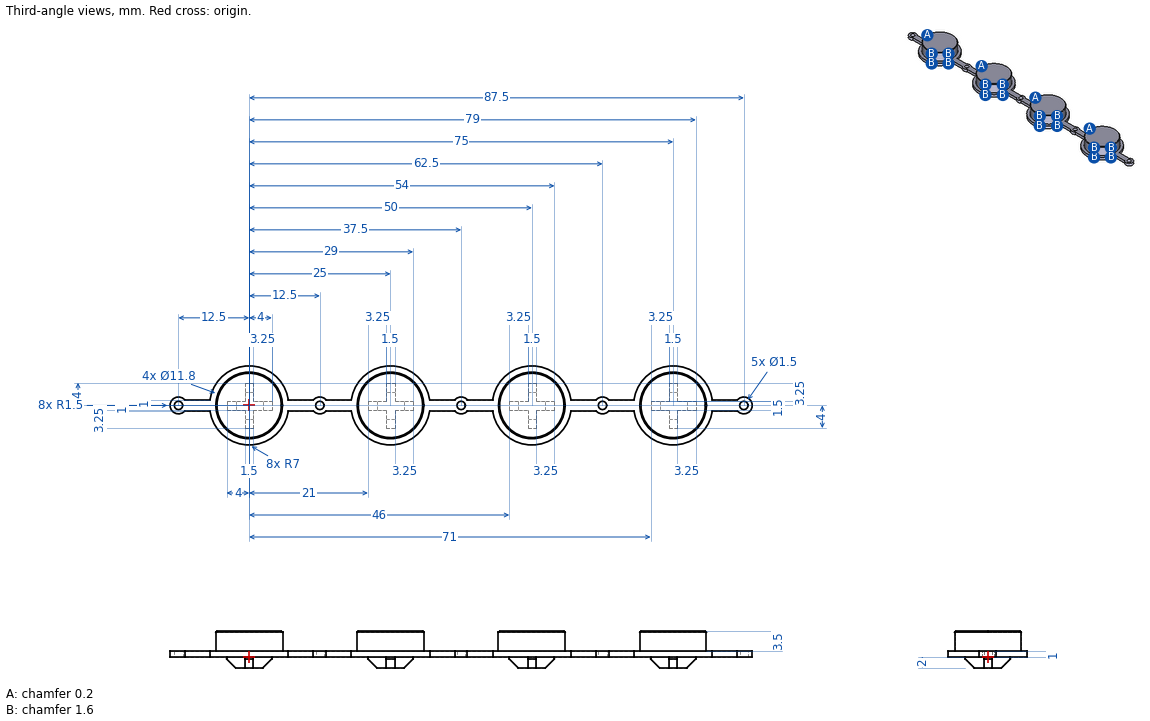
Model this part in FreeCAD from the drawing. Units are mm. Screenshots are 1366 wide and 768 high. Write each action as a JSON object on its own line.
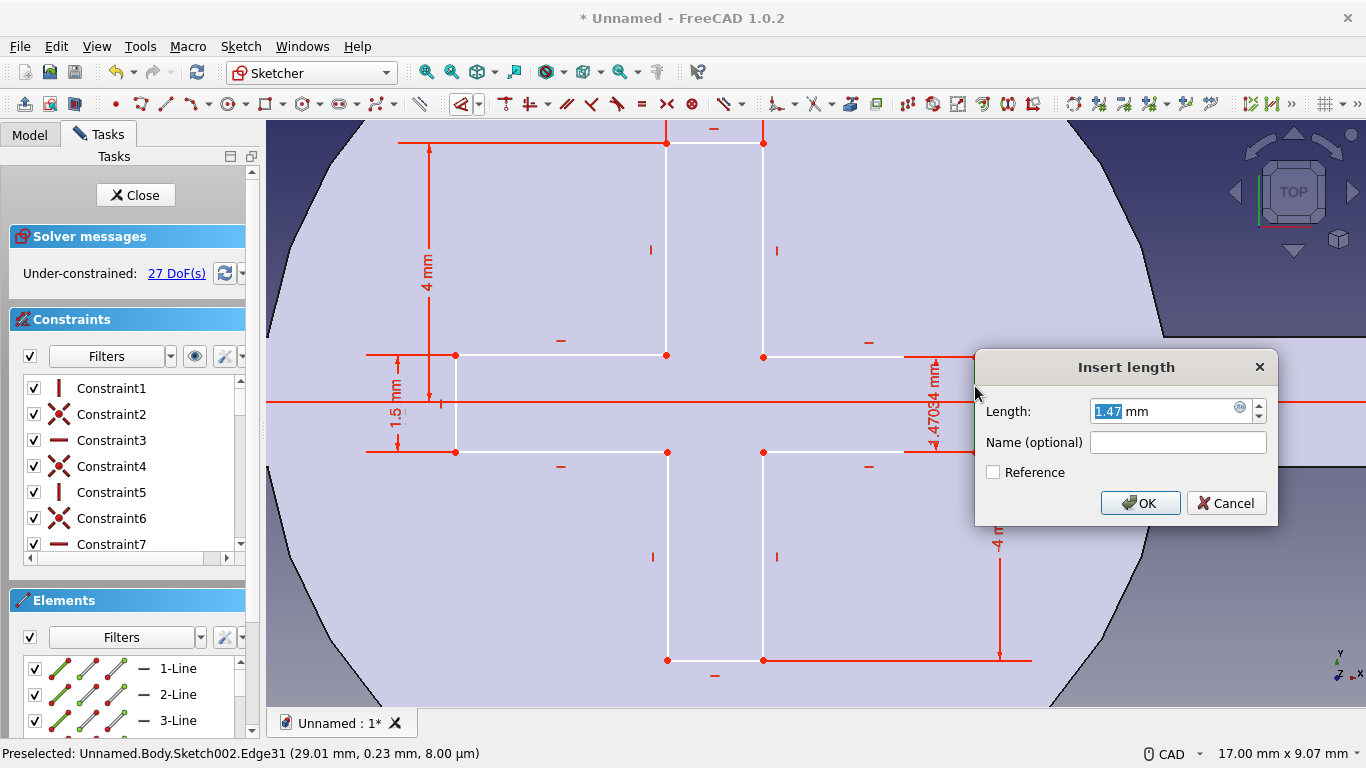
{"action": "type", "text": "1.5"}
{"action": "key", "text": "Return"}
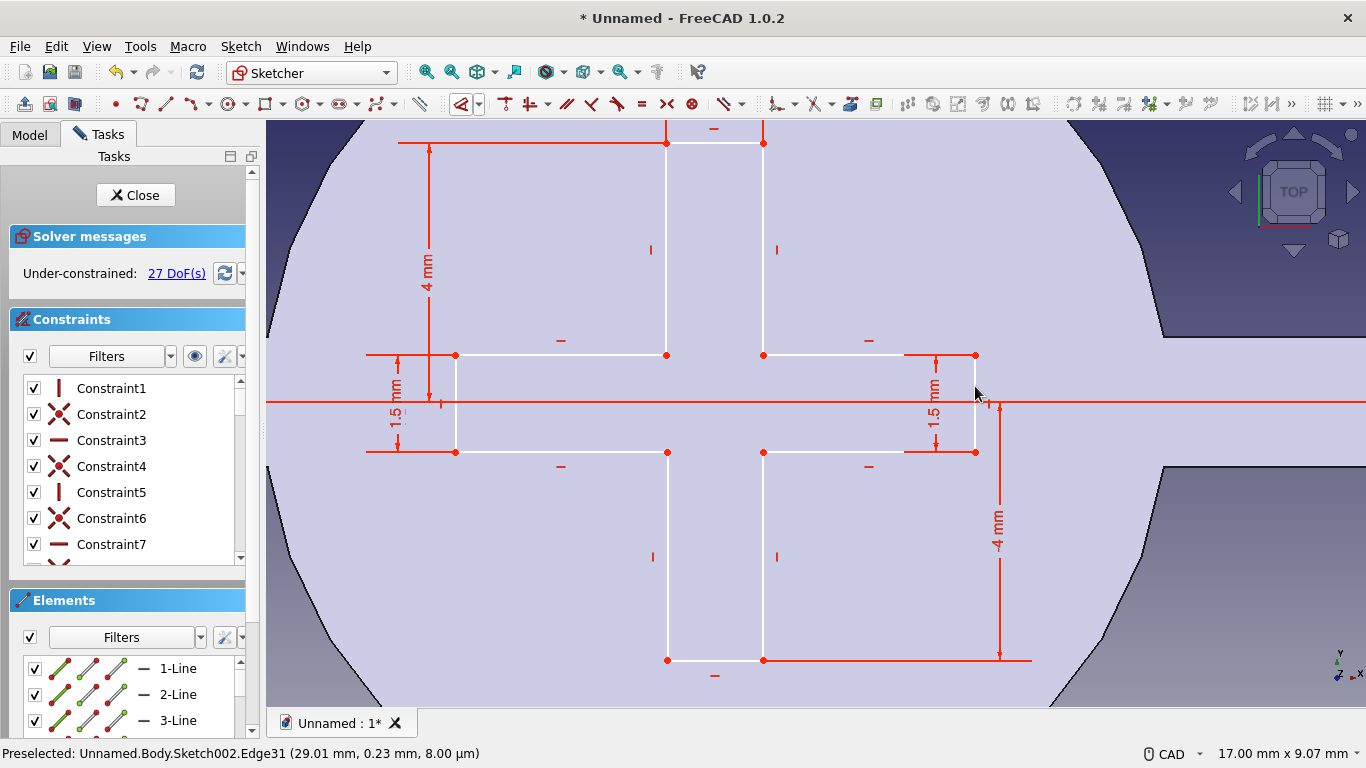
{"action": "left_click", "coordinate": [735, 661]}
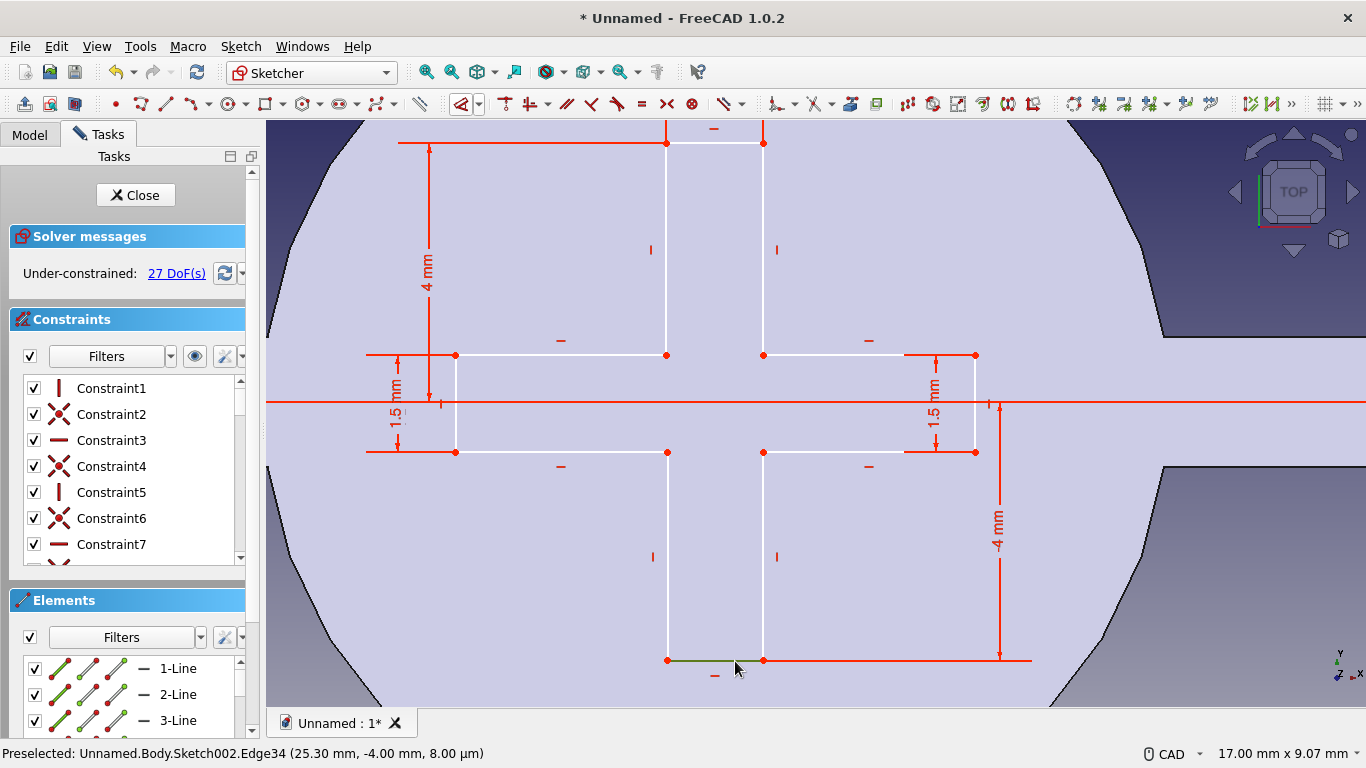
{"action": "key", "text": "l"}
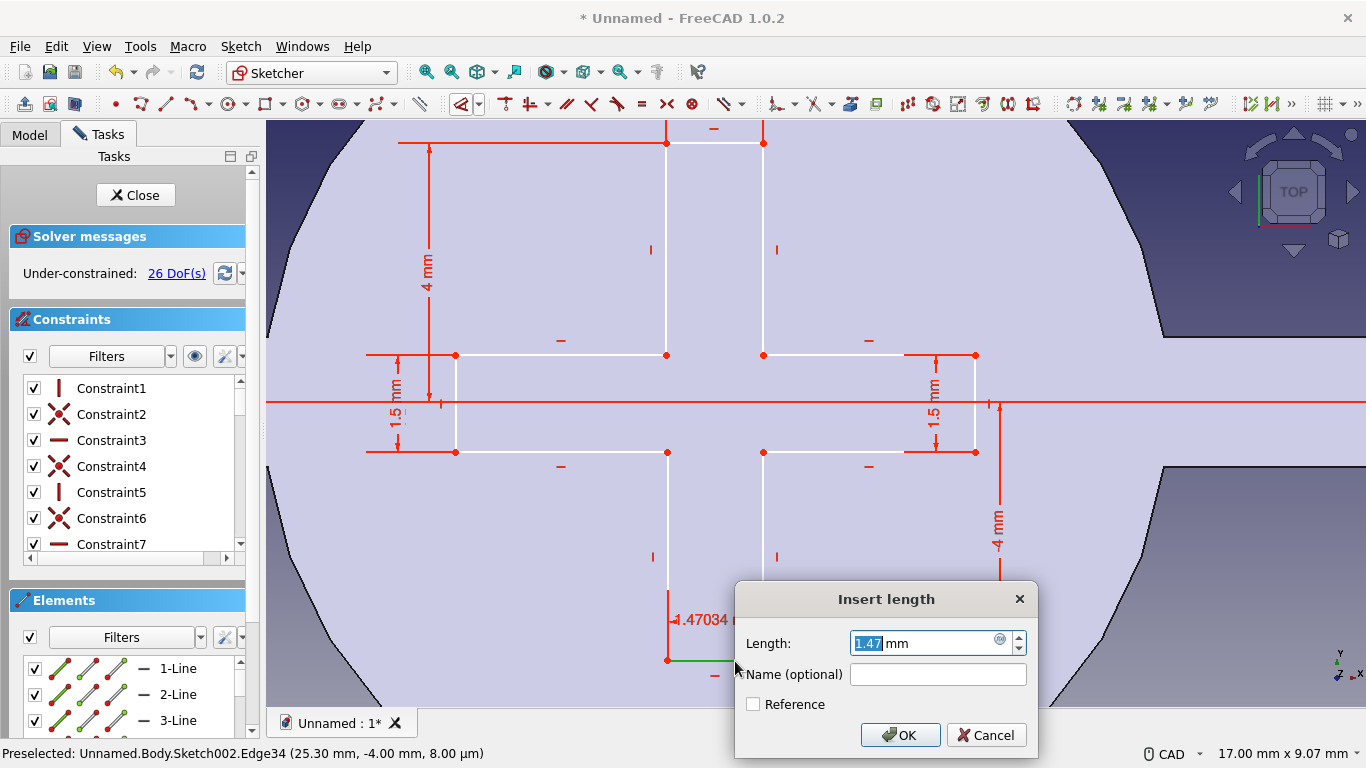
{"action": "type", "text": "1.5"}
{"action": "key", "text": "Return"}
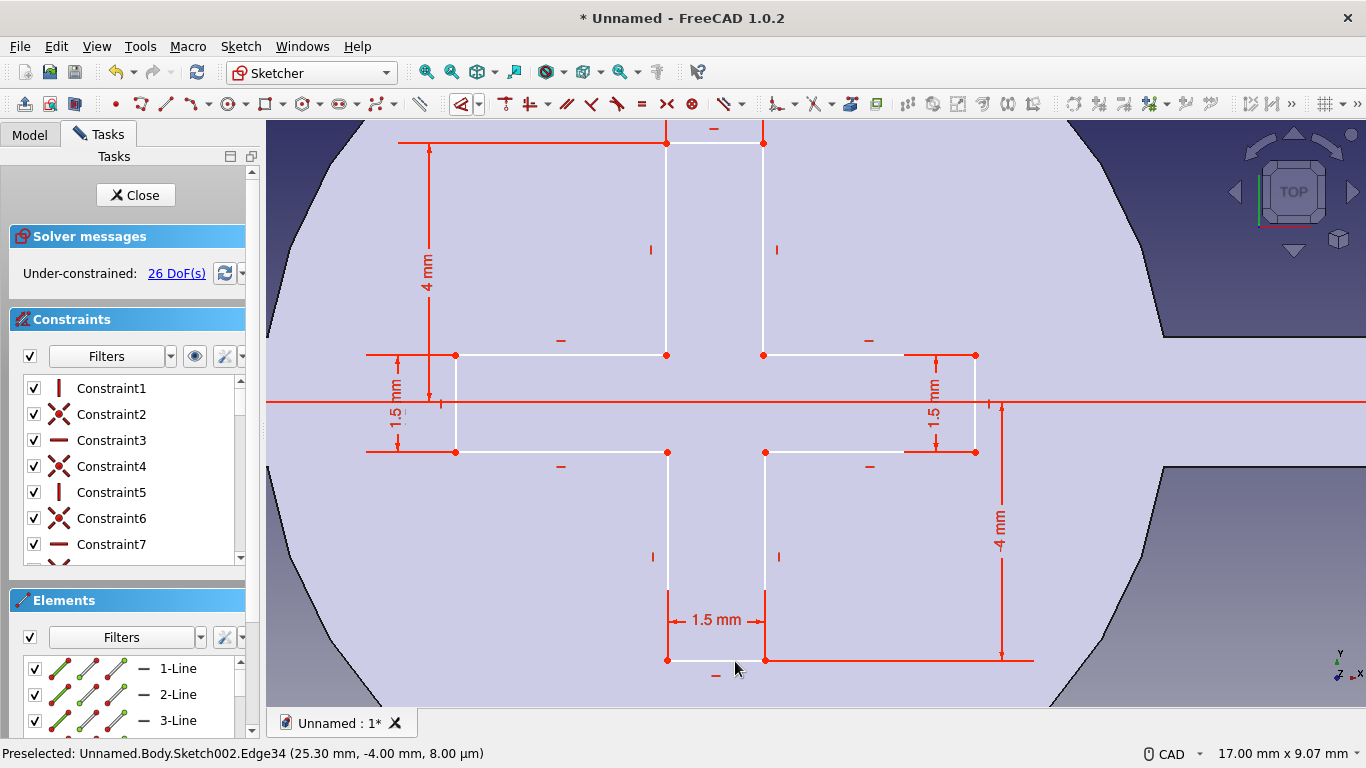
{"action": "scroll", "coordinate": [651, 415], "scroll_direction": "down", "scroll_amount": 11}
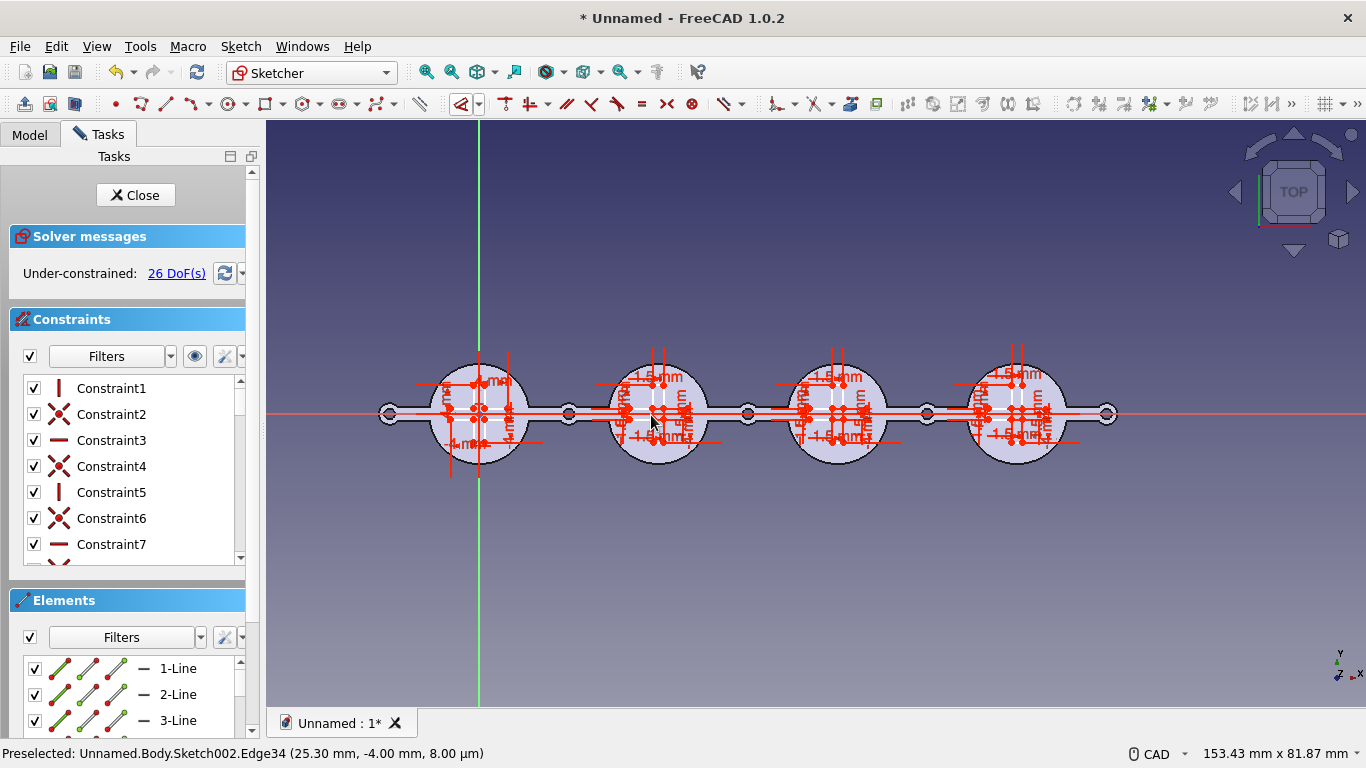
{"action": "scroll", "coordinate": [508, 412], "scroll_direction": "up", "scroll_amount": 10}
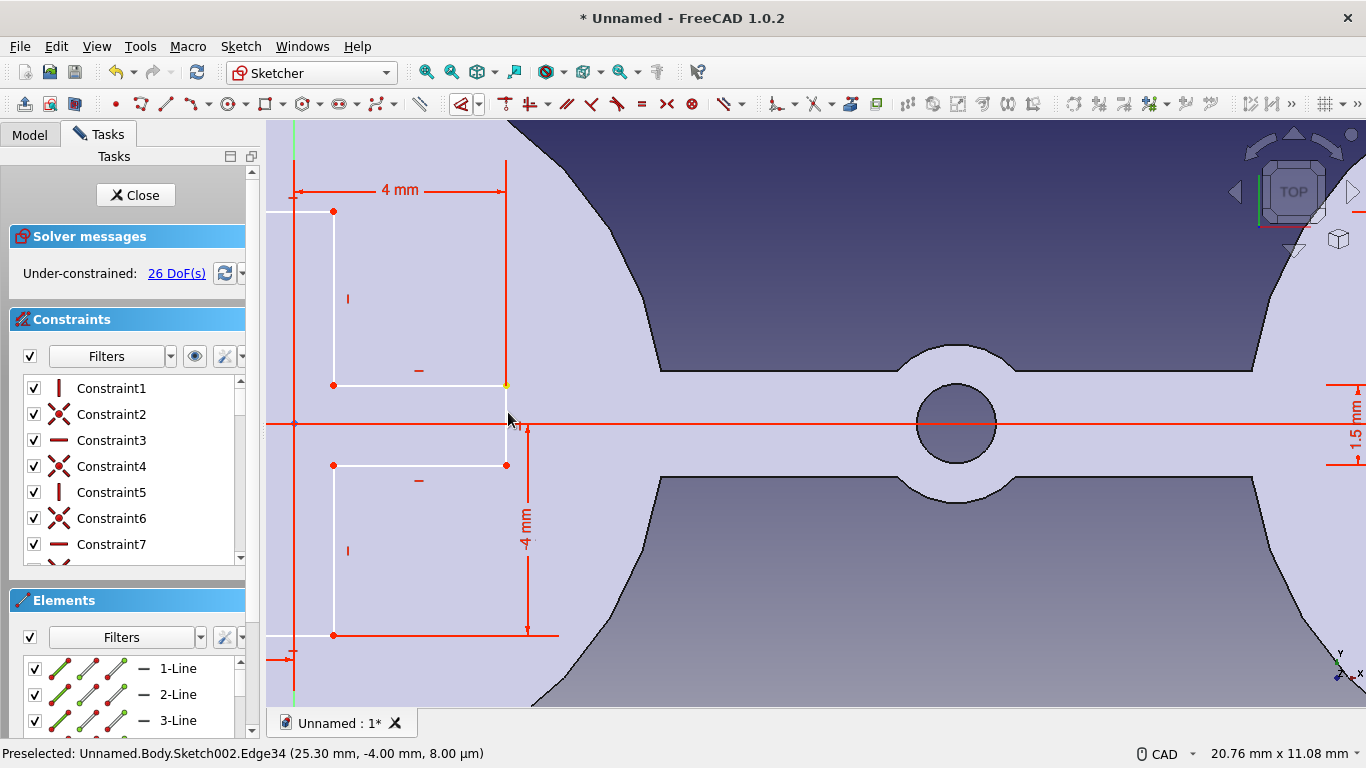
{"action": "left_click", "coordinate": [506, 410]}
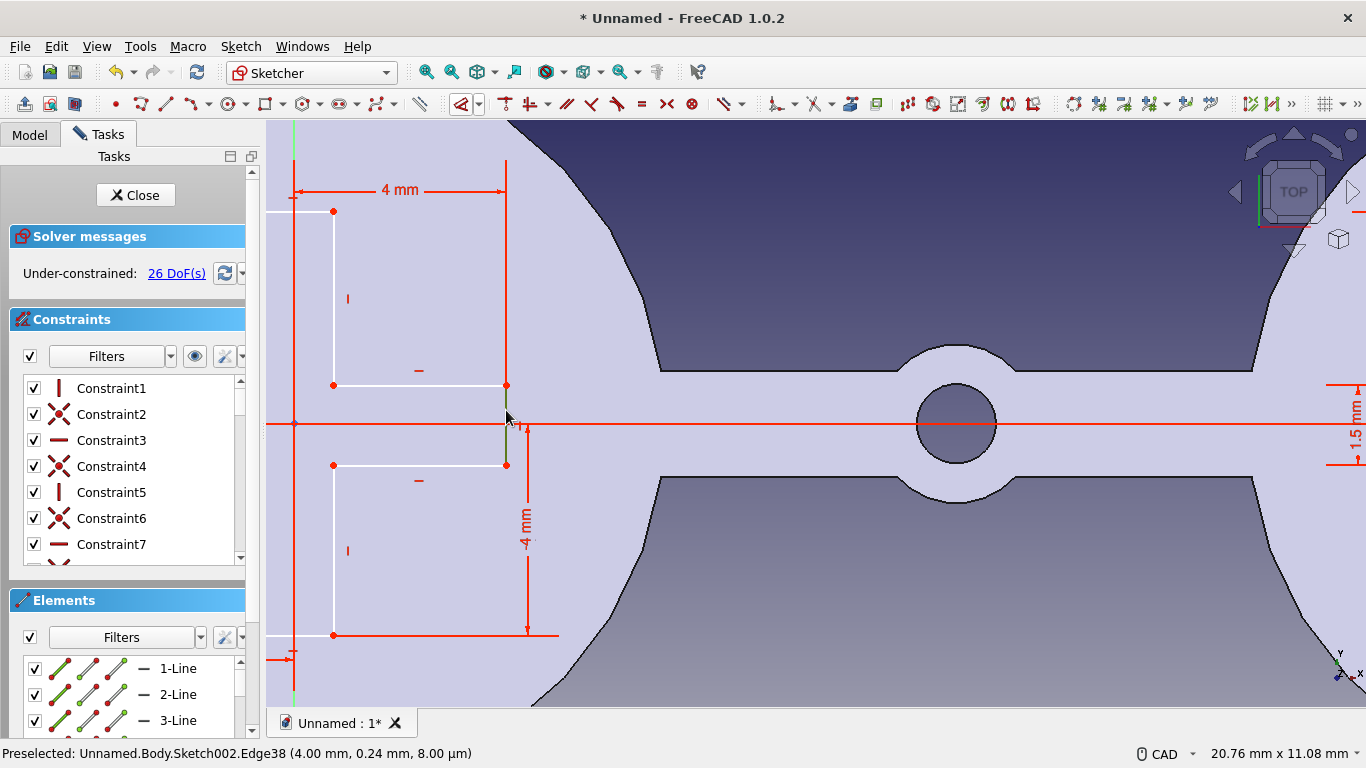
{"action": "left_click", "coordinate": [478, 104]}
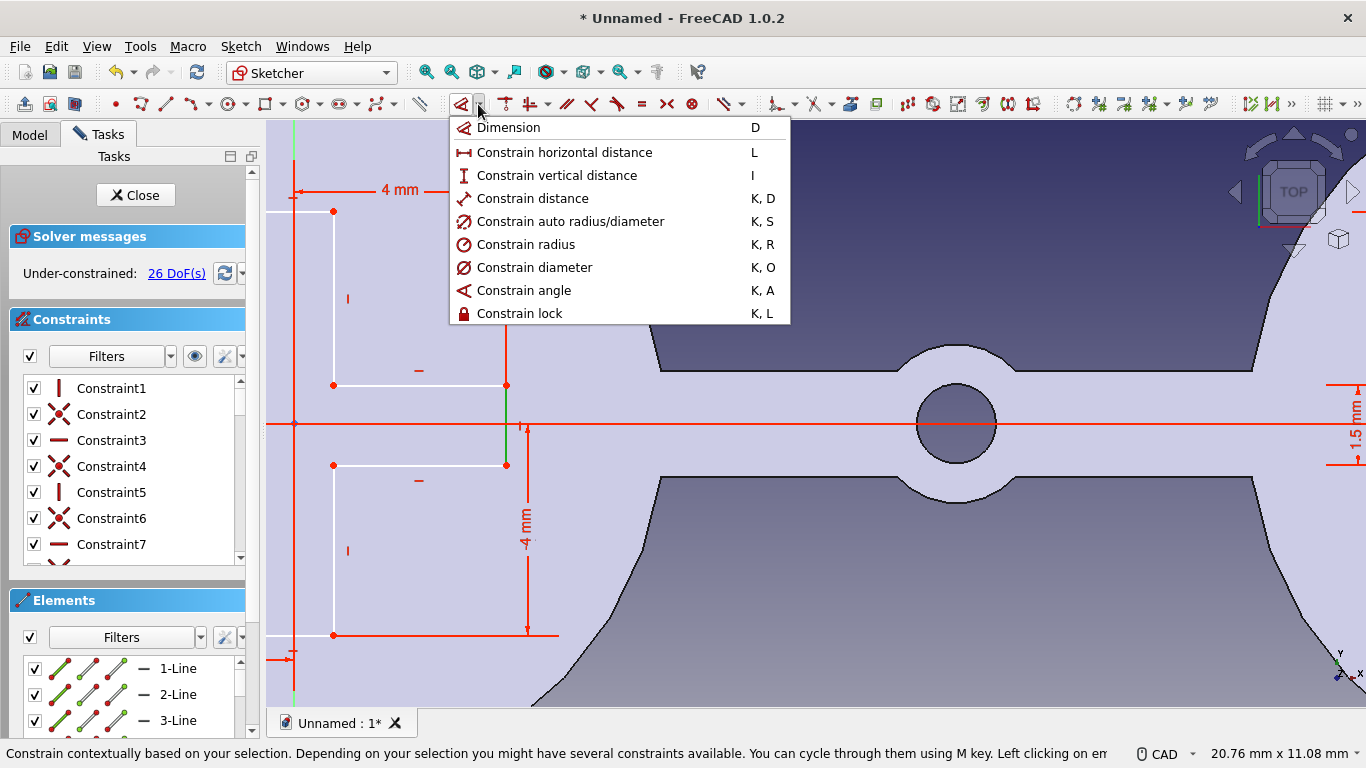
{"action": "left_click", "coordinate": [620, 176]}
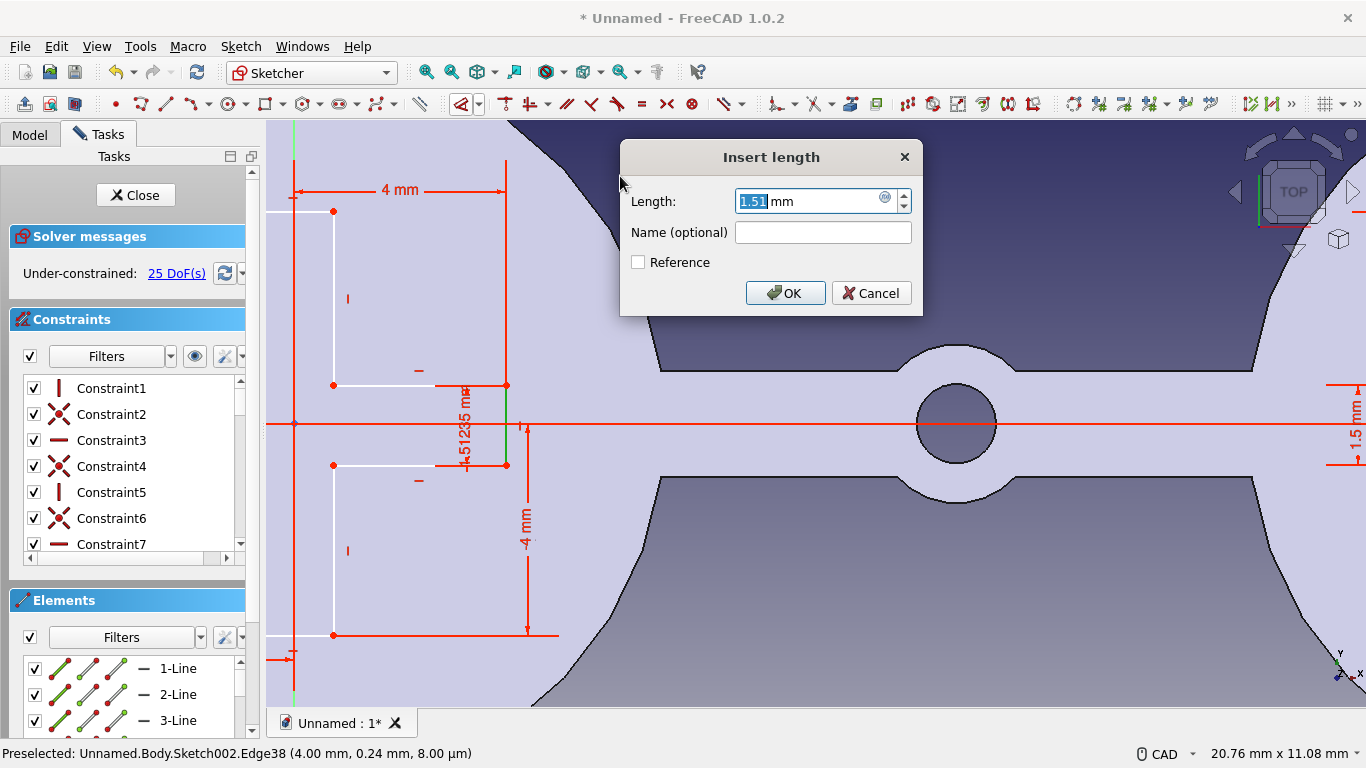
{"action": "type", "text": "1.5"}
{"action": "key", "text": "Return"}